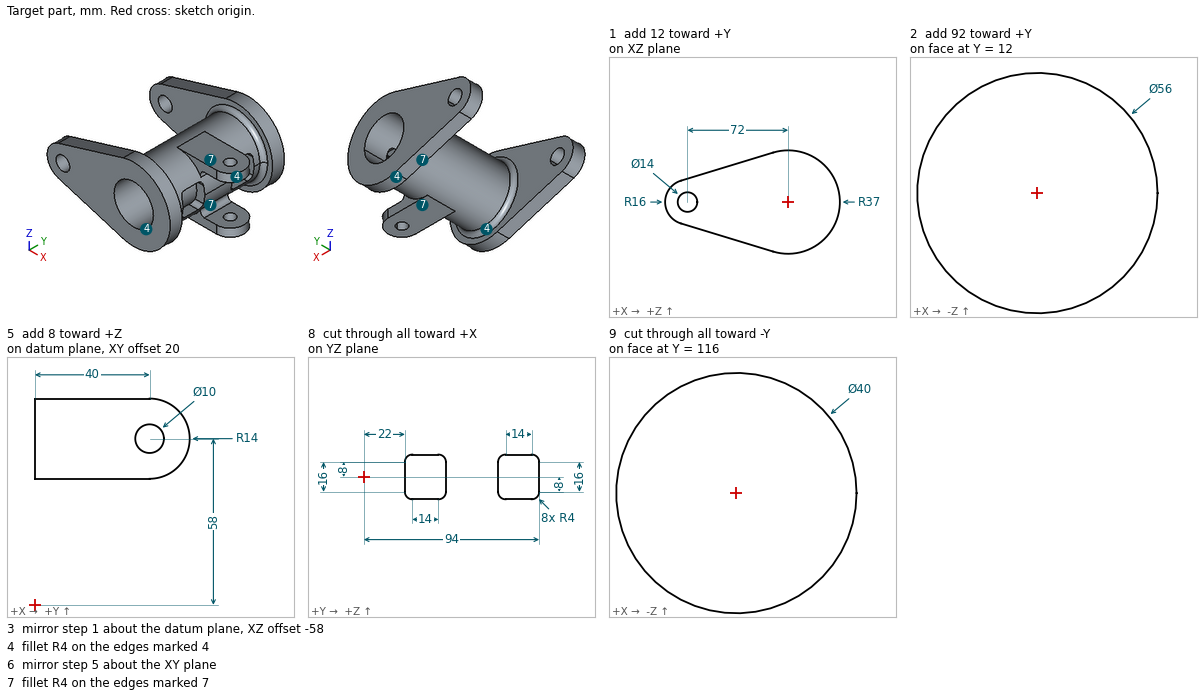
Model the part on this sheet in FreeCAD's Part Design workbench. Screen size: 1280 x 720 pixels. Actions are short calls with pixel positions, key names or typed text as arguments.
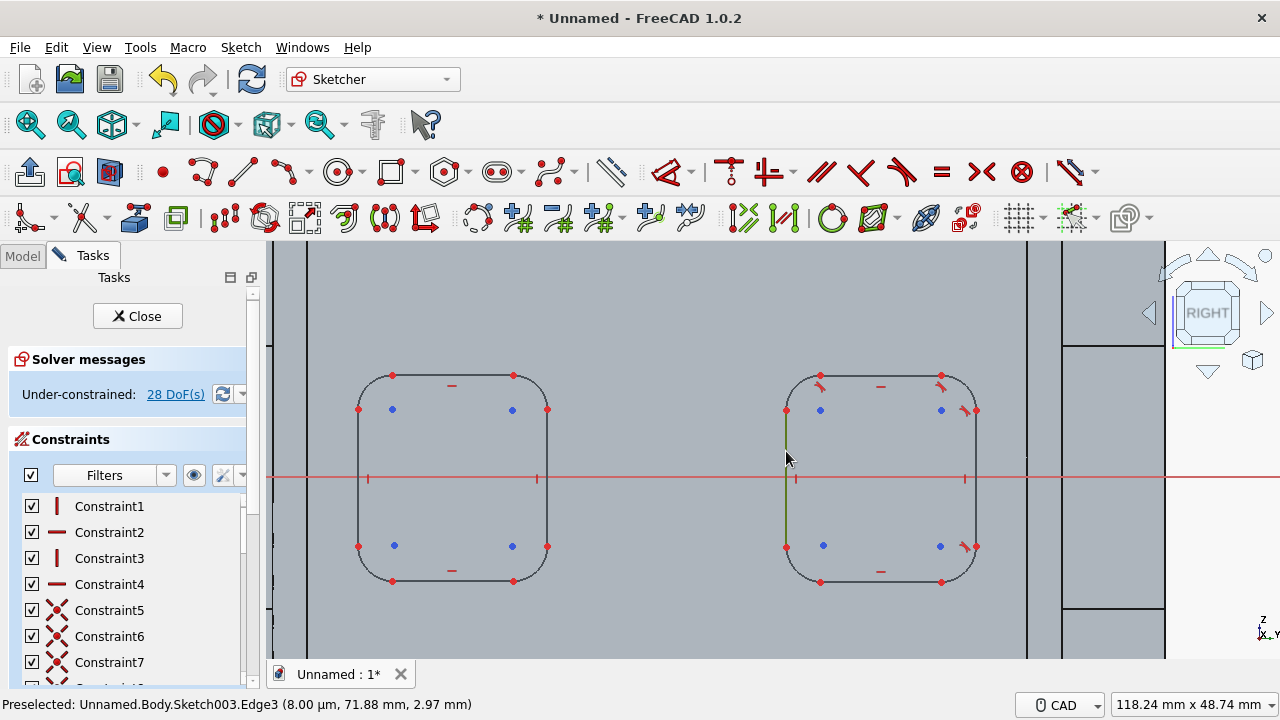
click(805, 379)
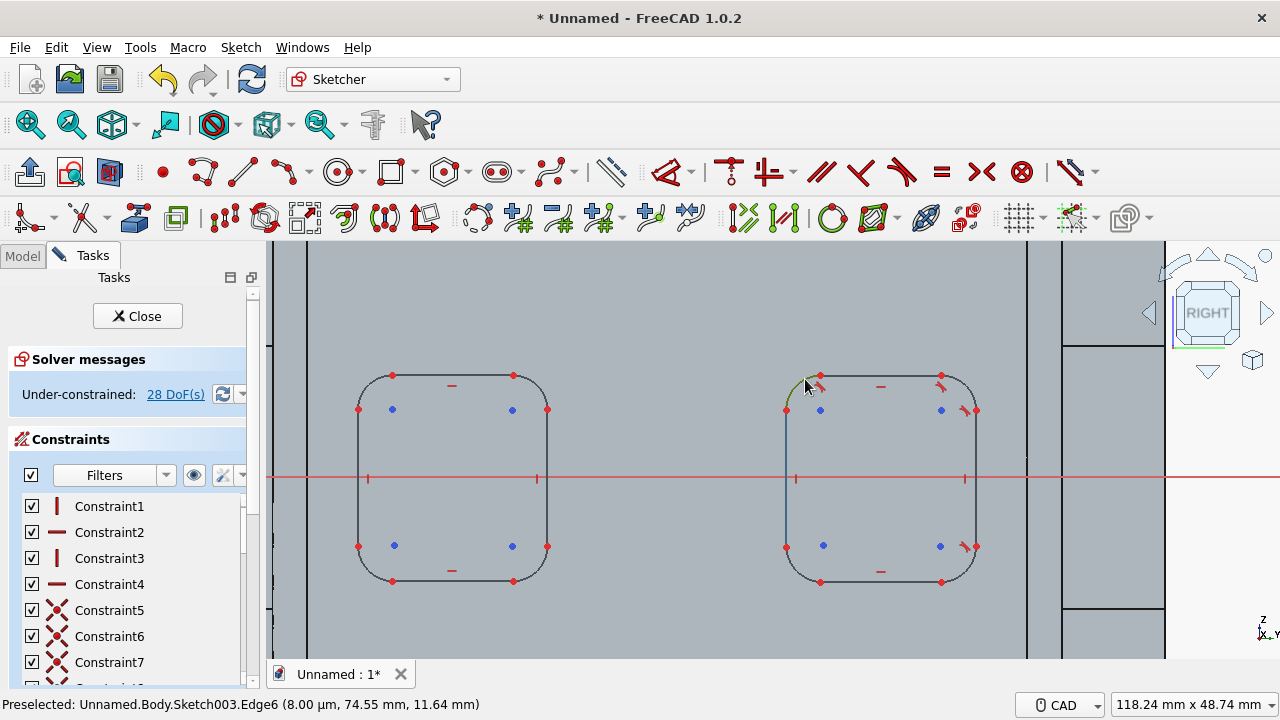
key(t)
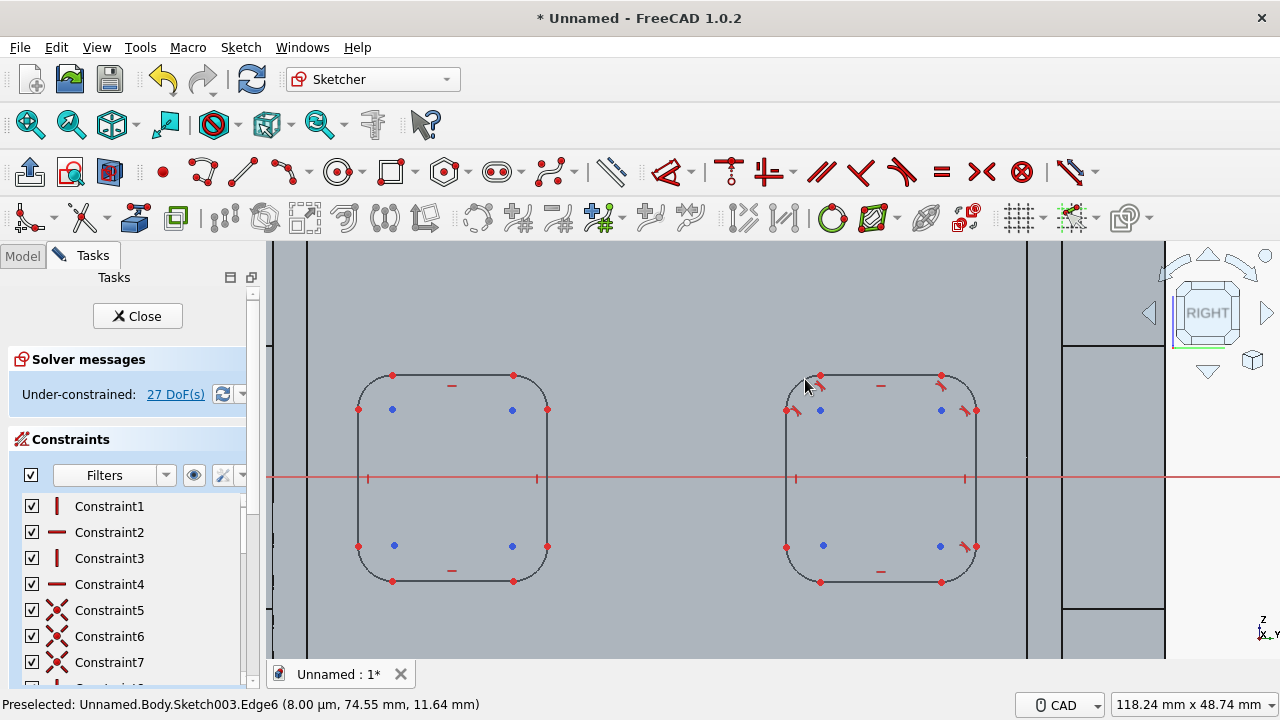
click(786, 451)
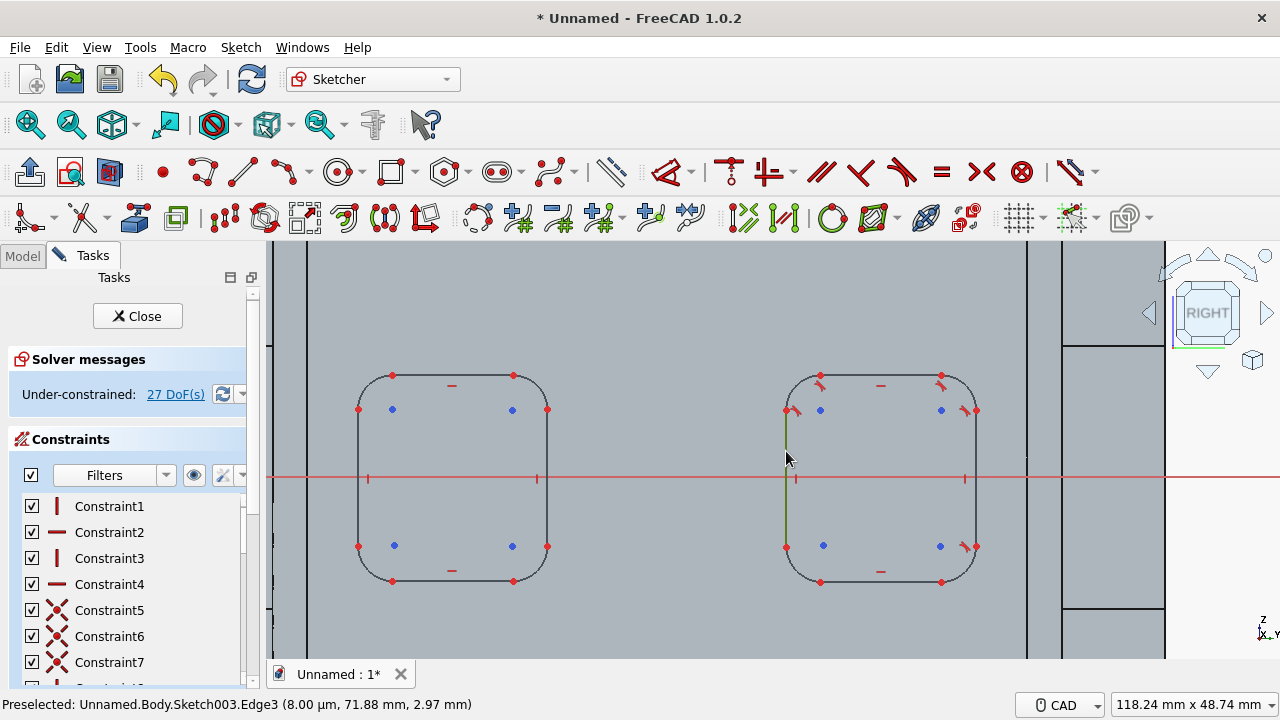
click(791, 563)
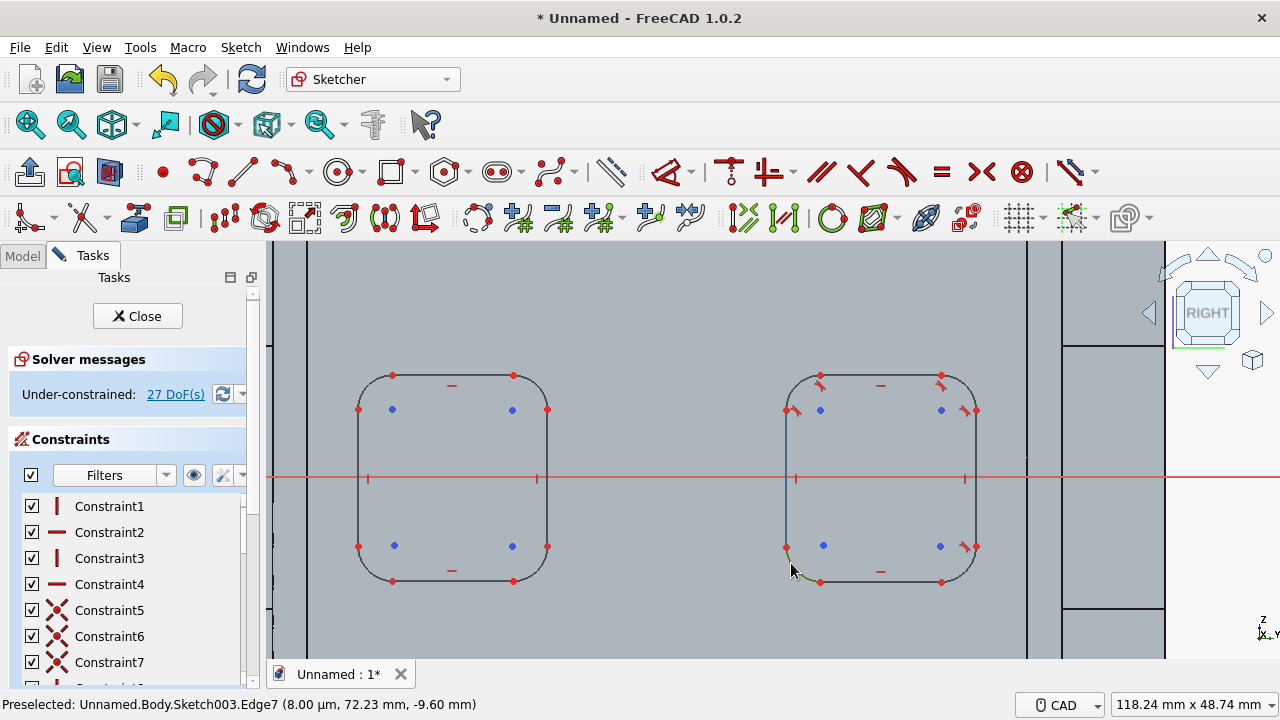
key(t)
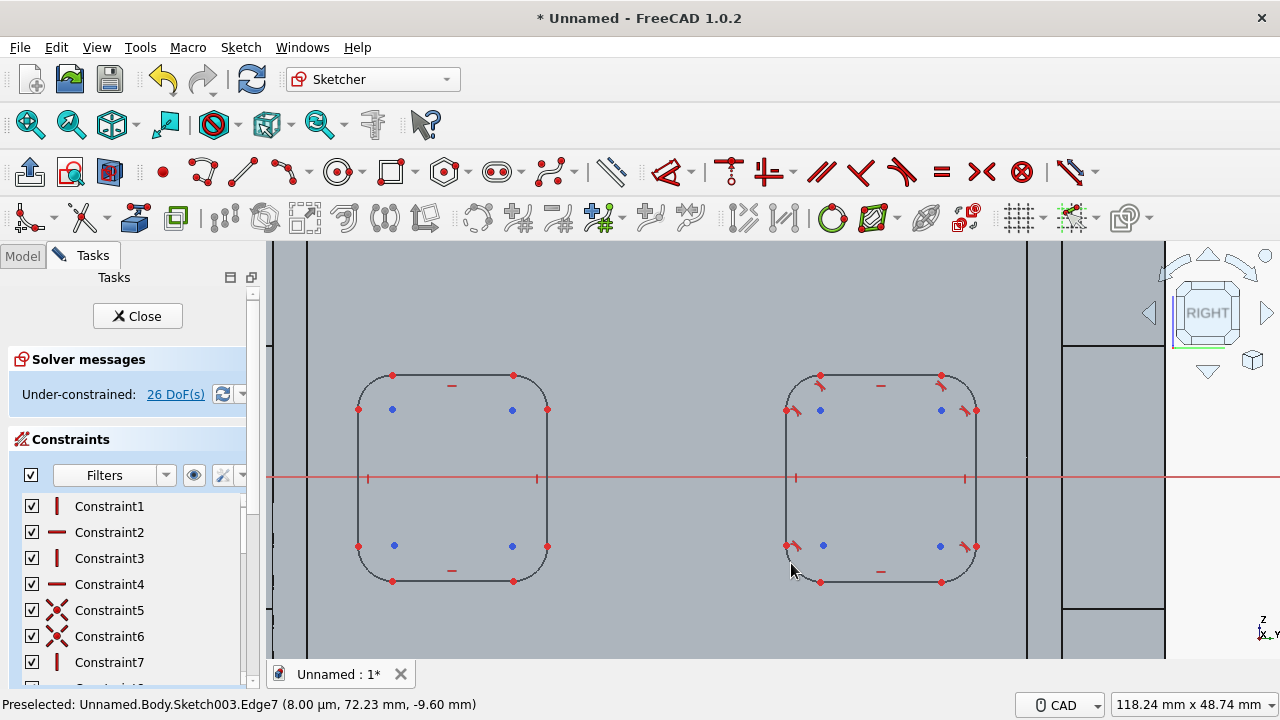
click(857, 582)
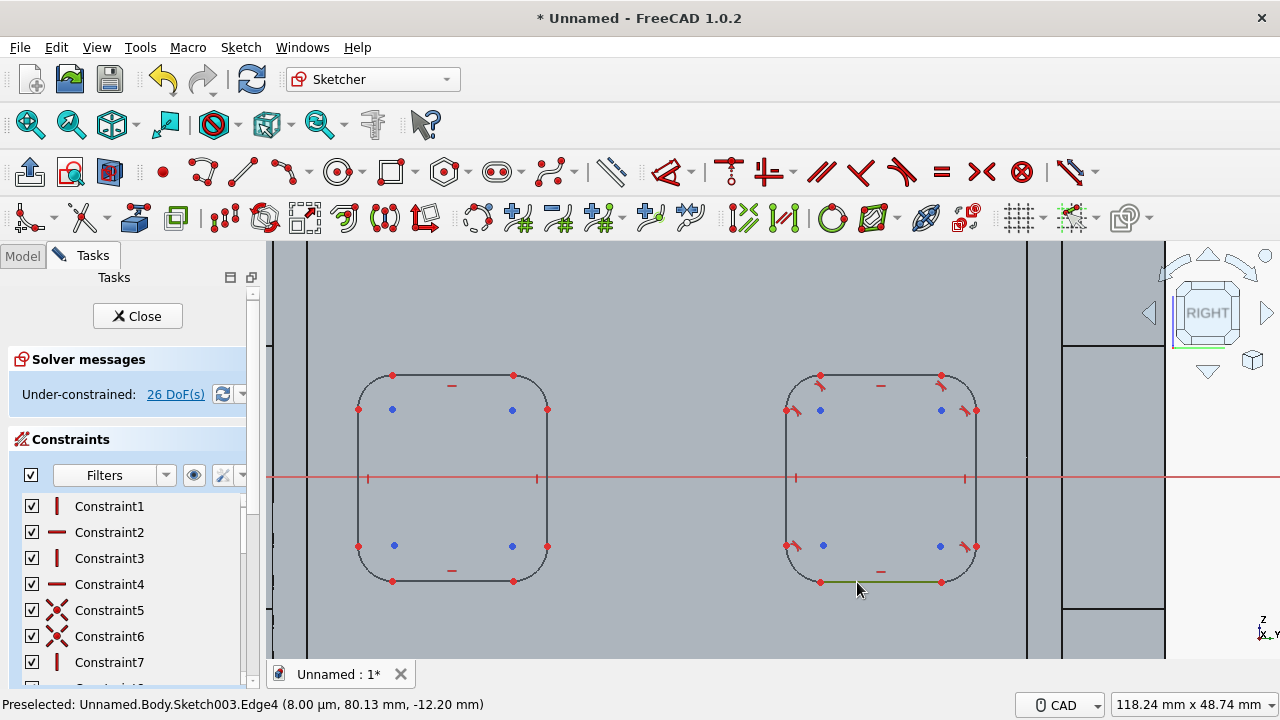
click(790, 561)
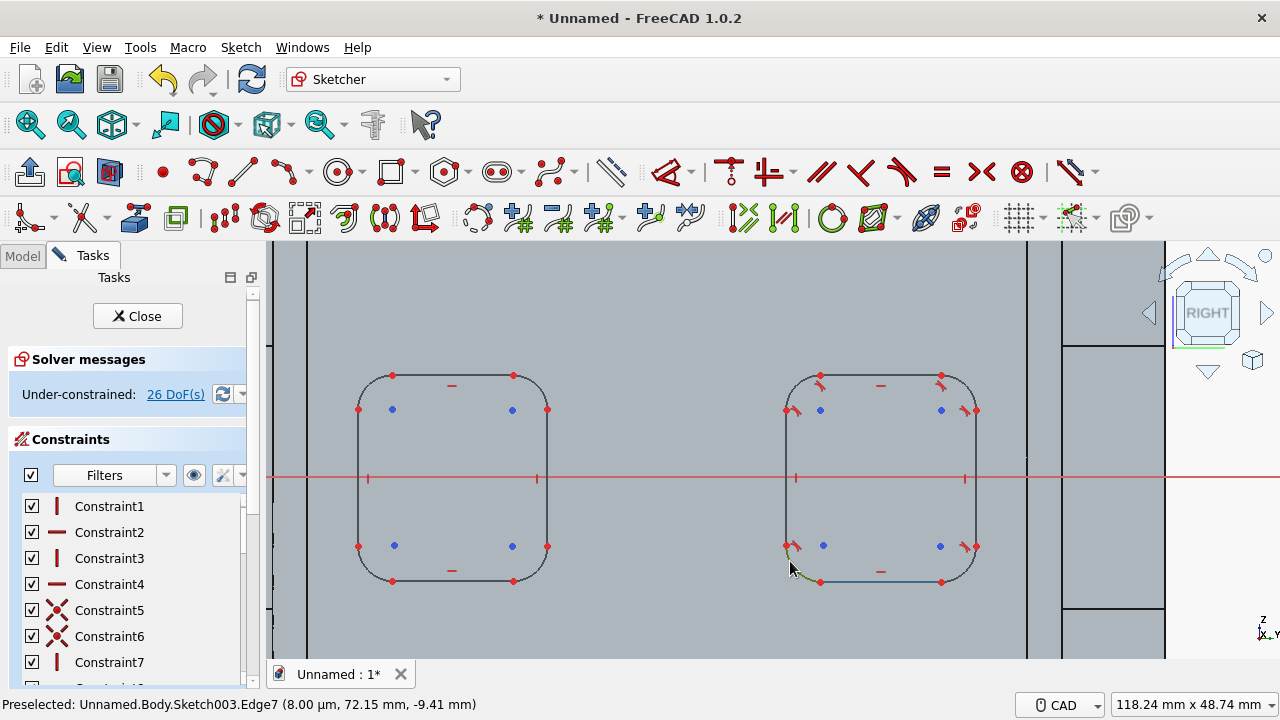
key(t)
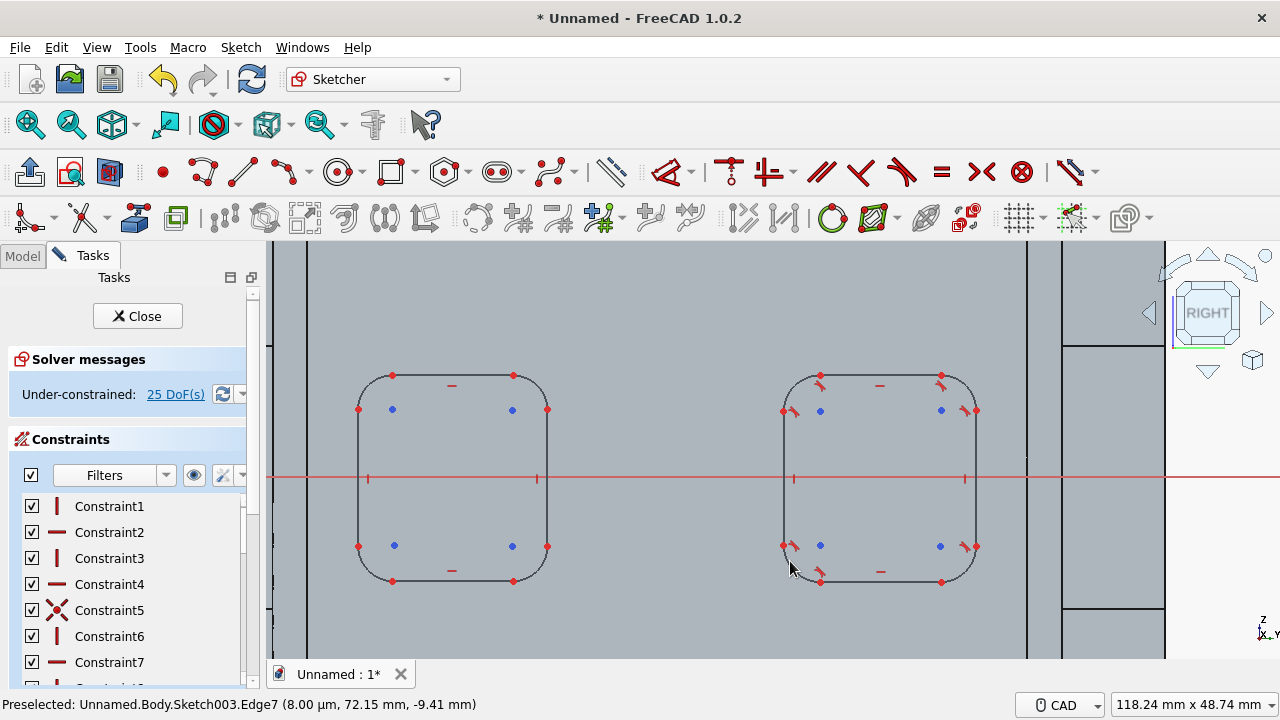
click(857, 582)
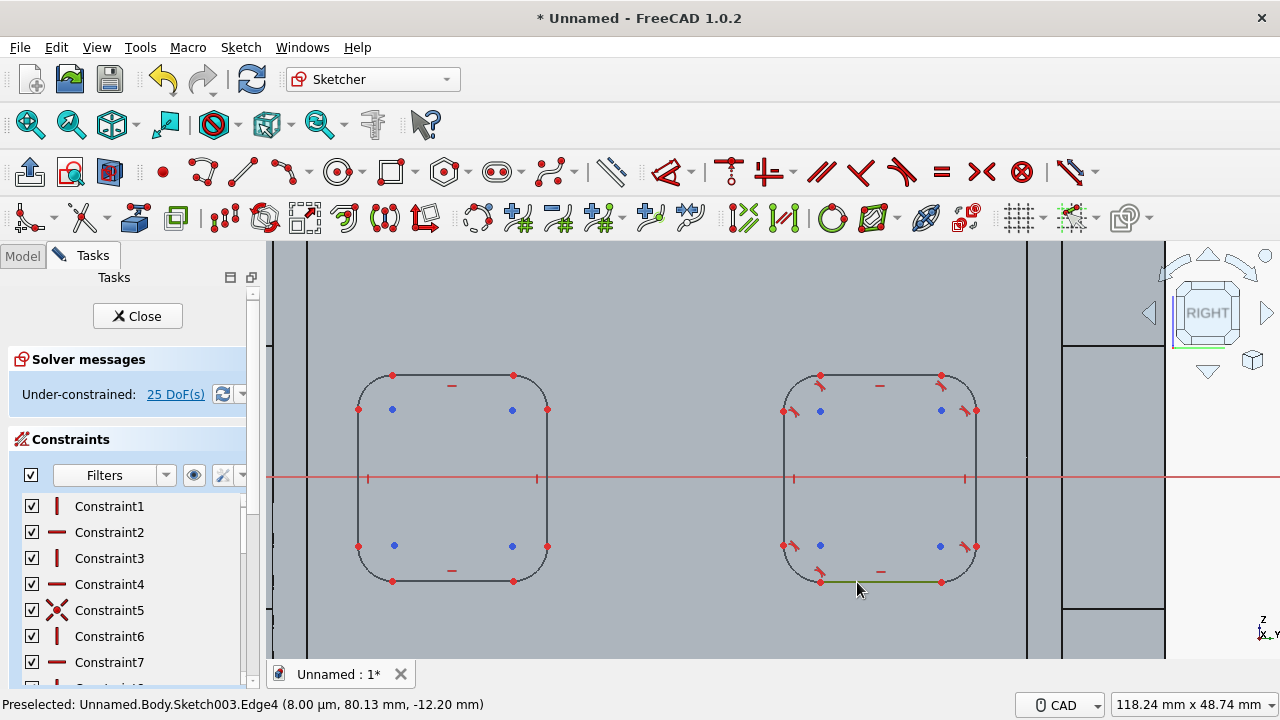
click(957, 578)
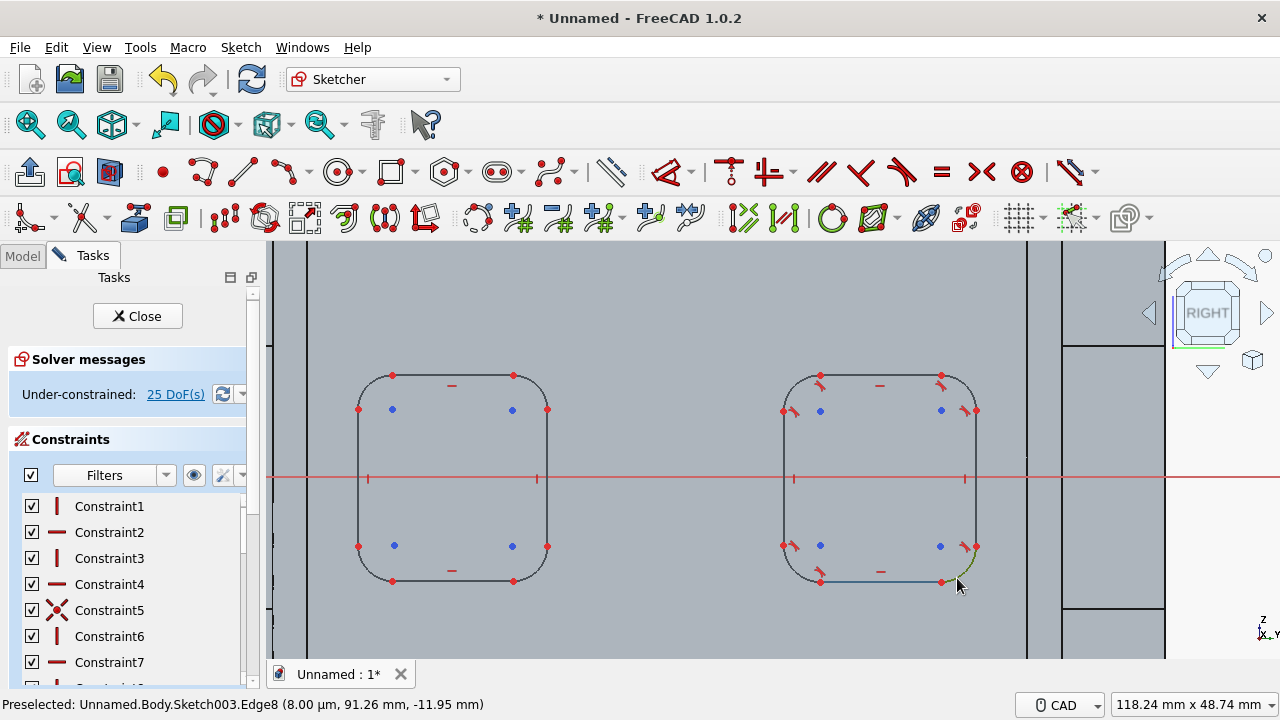
click(902, 172)